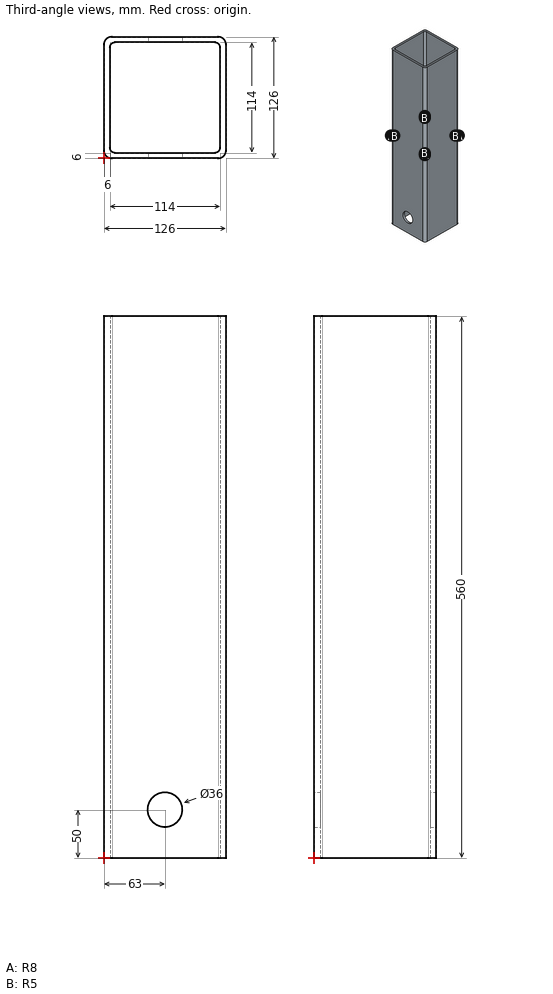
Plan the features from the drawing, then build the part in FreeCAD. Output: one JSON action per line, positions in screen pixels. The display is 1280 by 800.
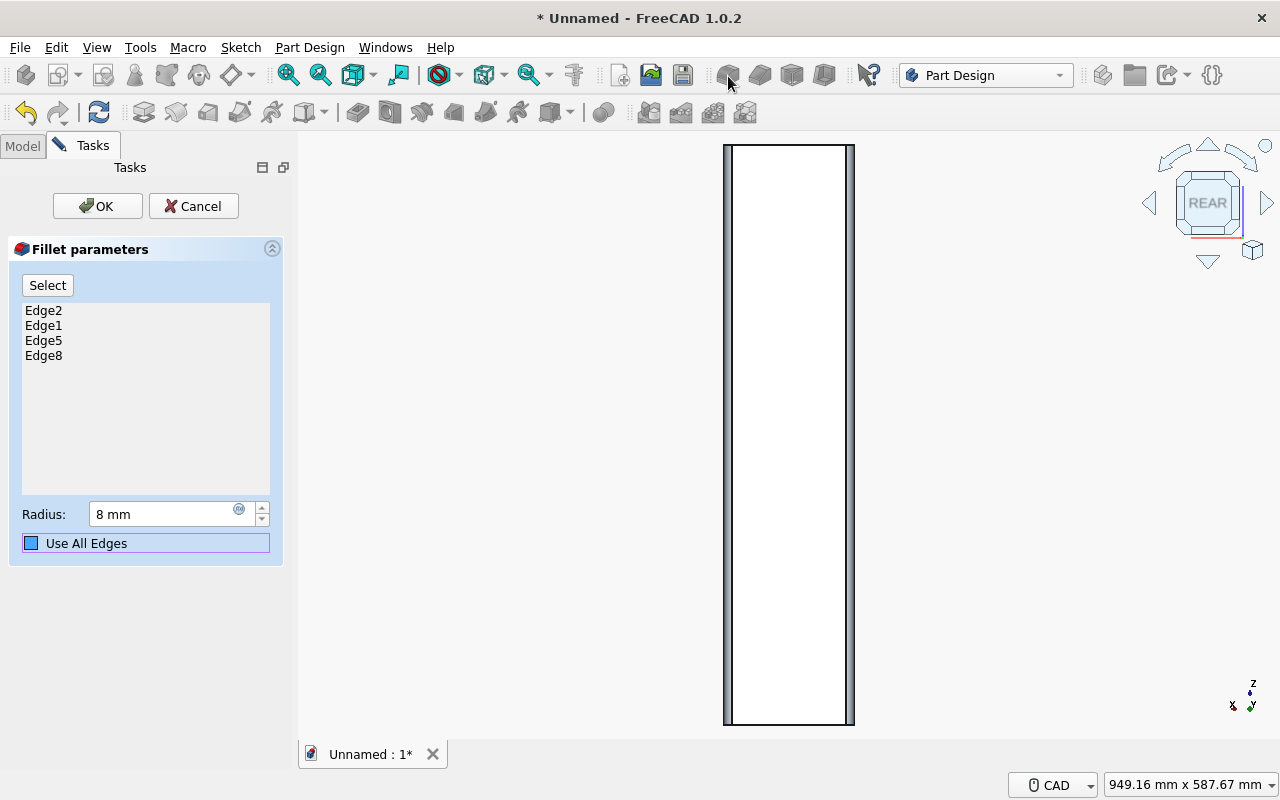
{"action": "left_click", "coordinate": [98, 206]}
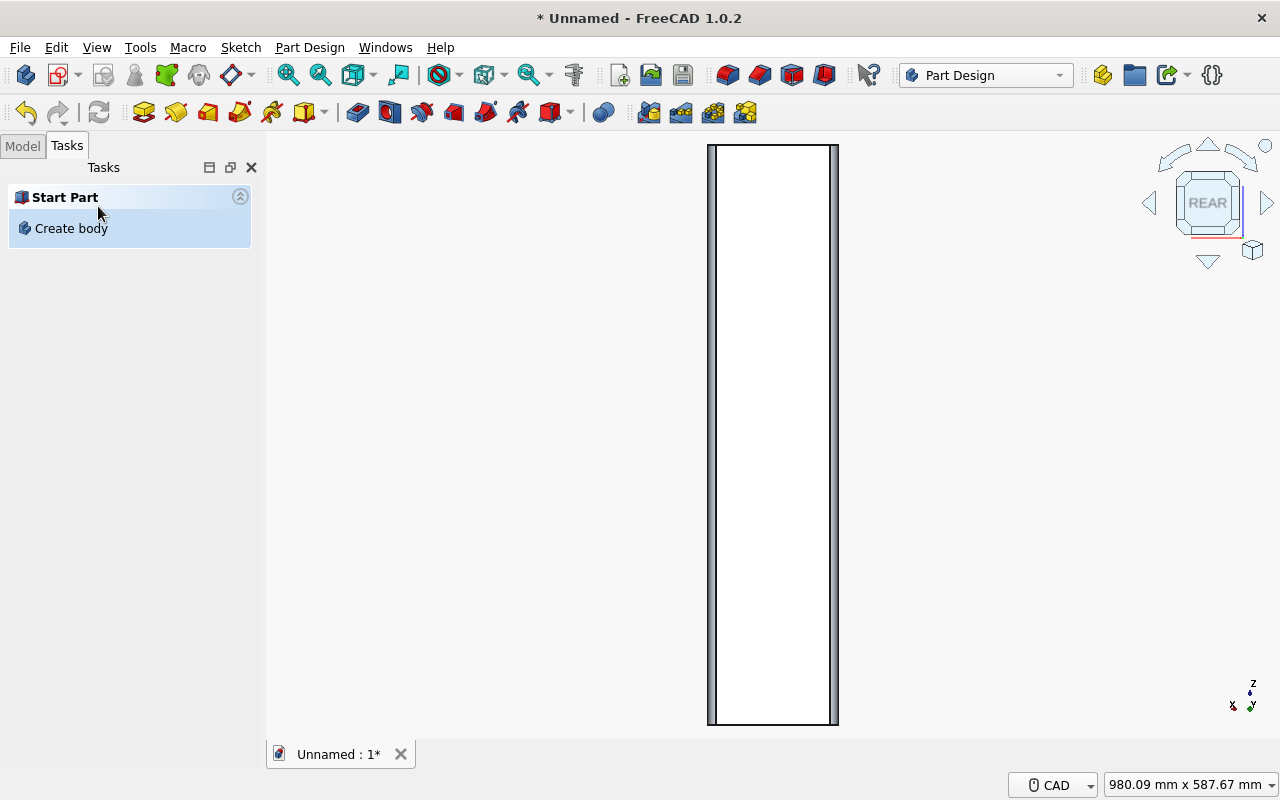
{"action": "key", "text": "0"}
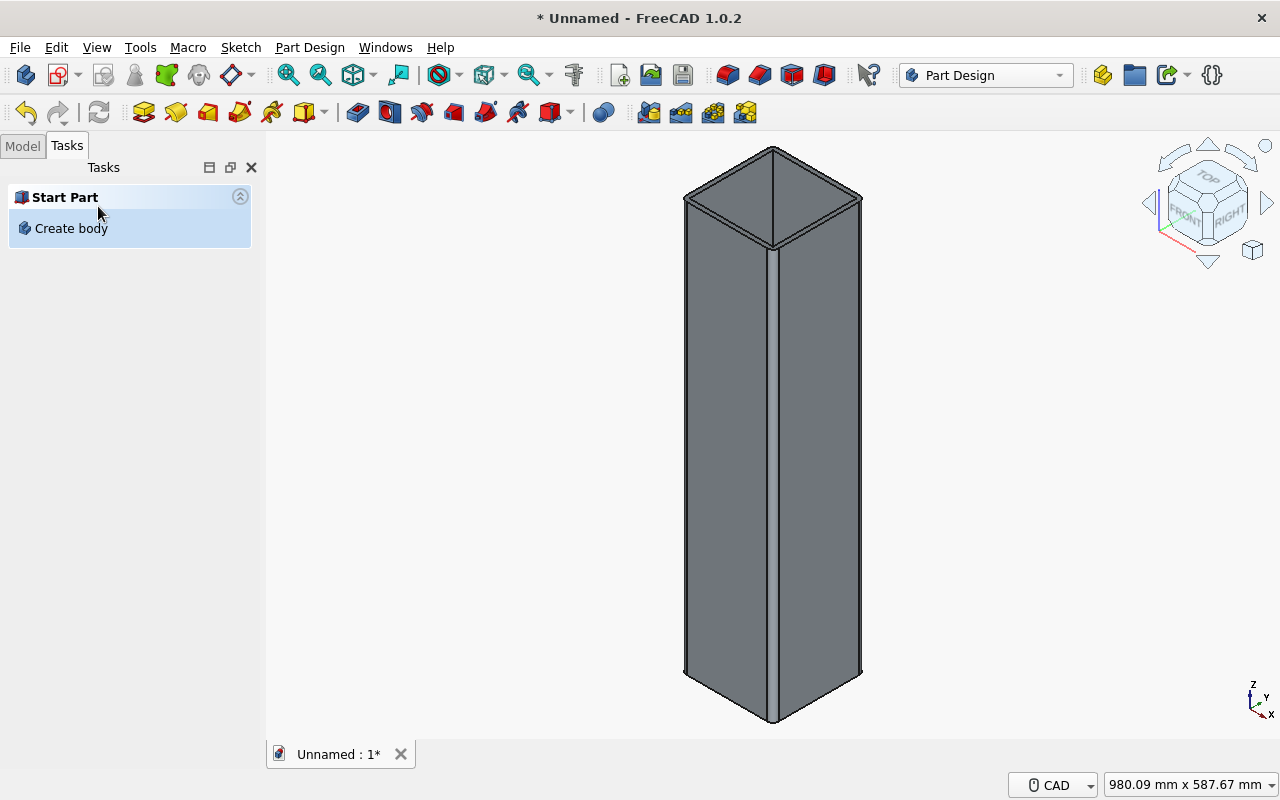
{"action": "key", "text": "2"}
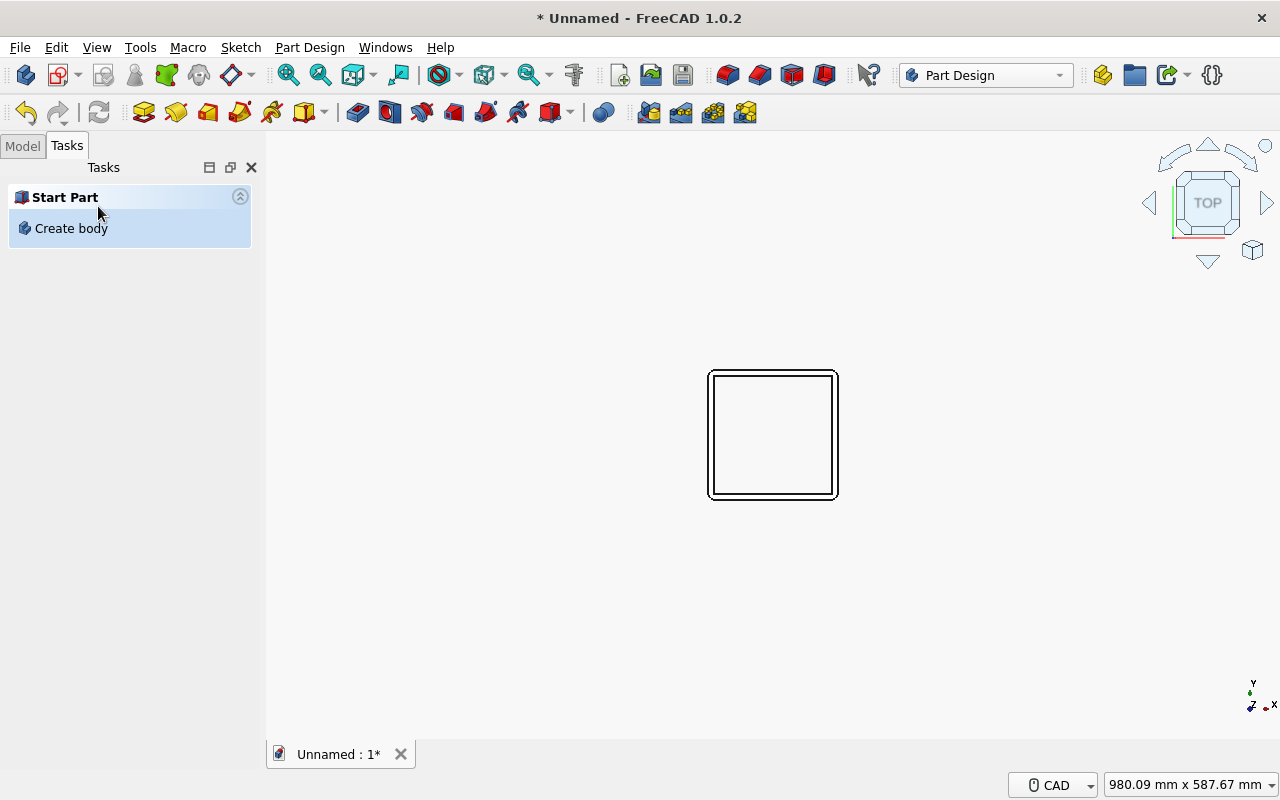
{"action": "left_click", "coordinate": [290, 76]}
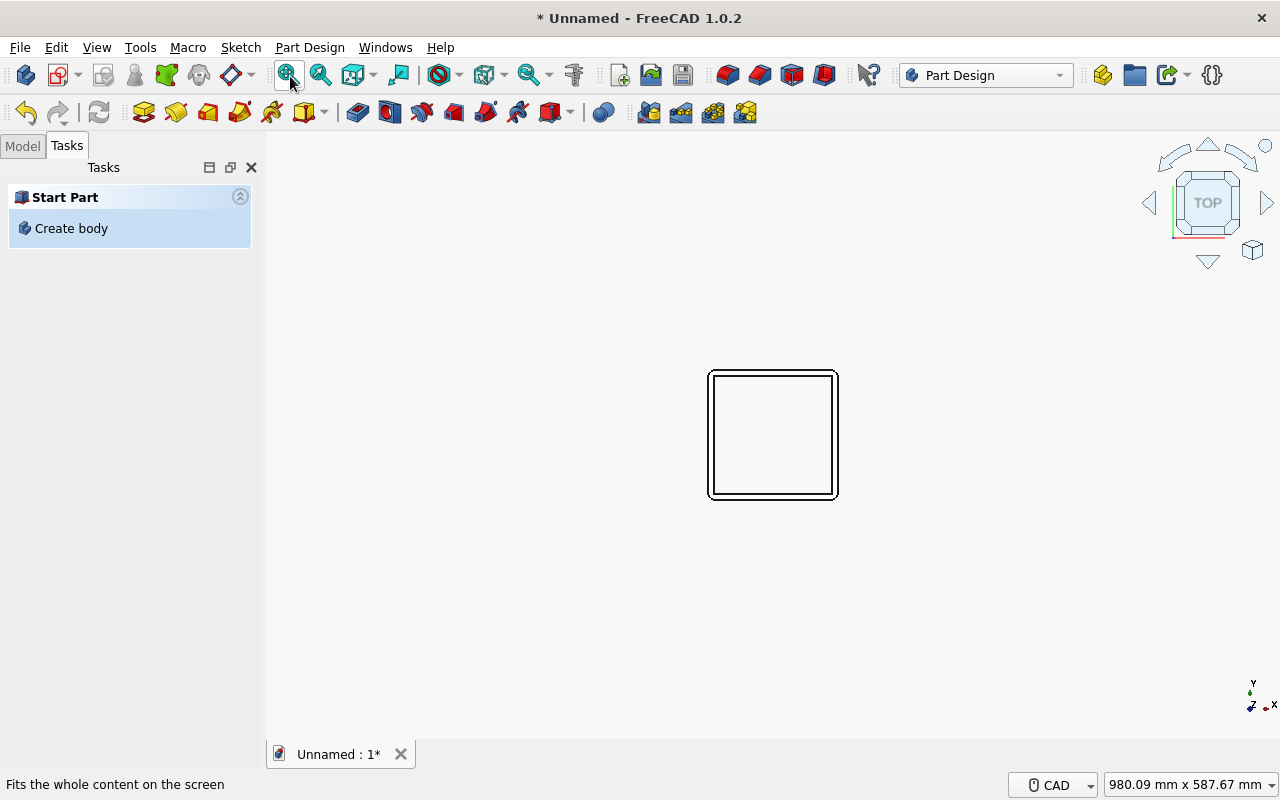
{"action": "key", "text": "1"}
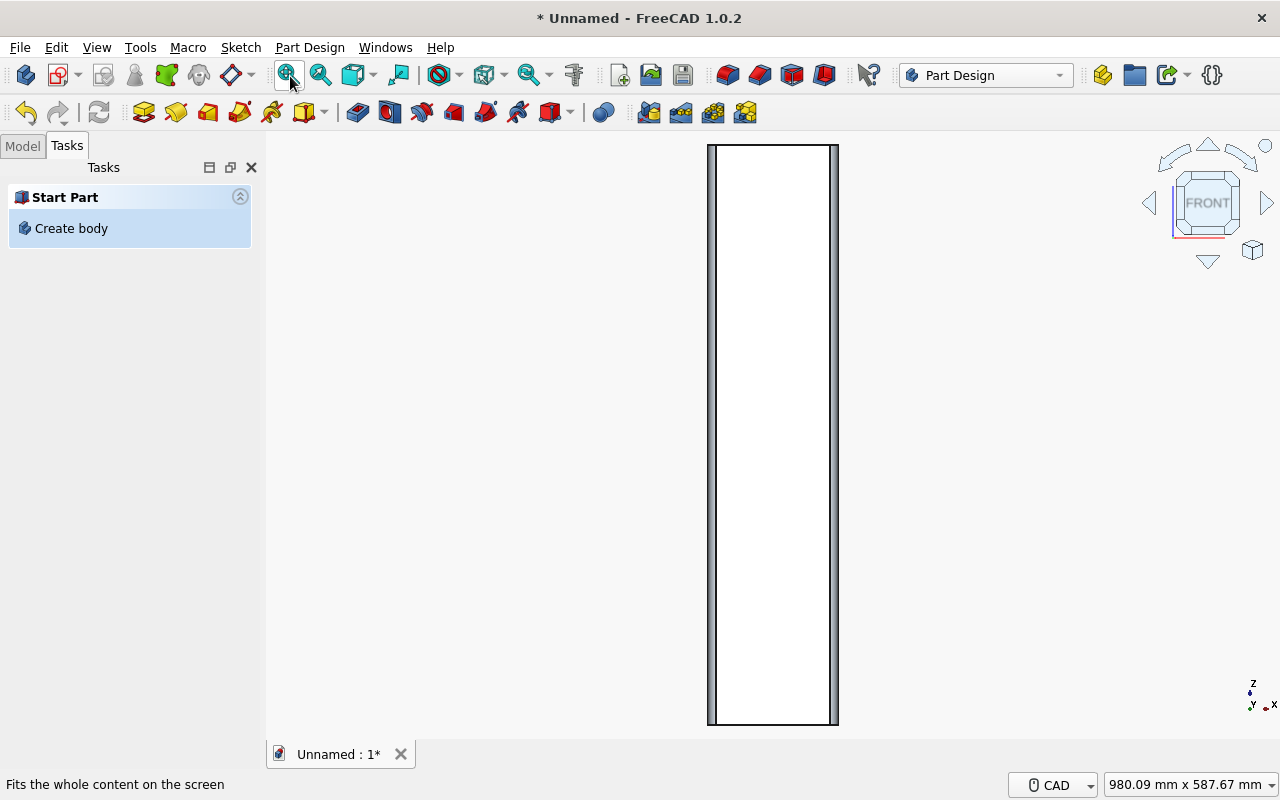
{"action": "key", "text": "3"}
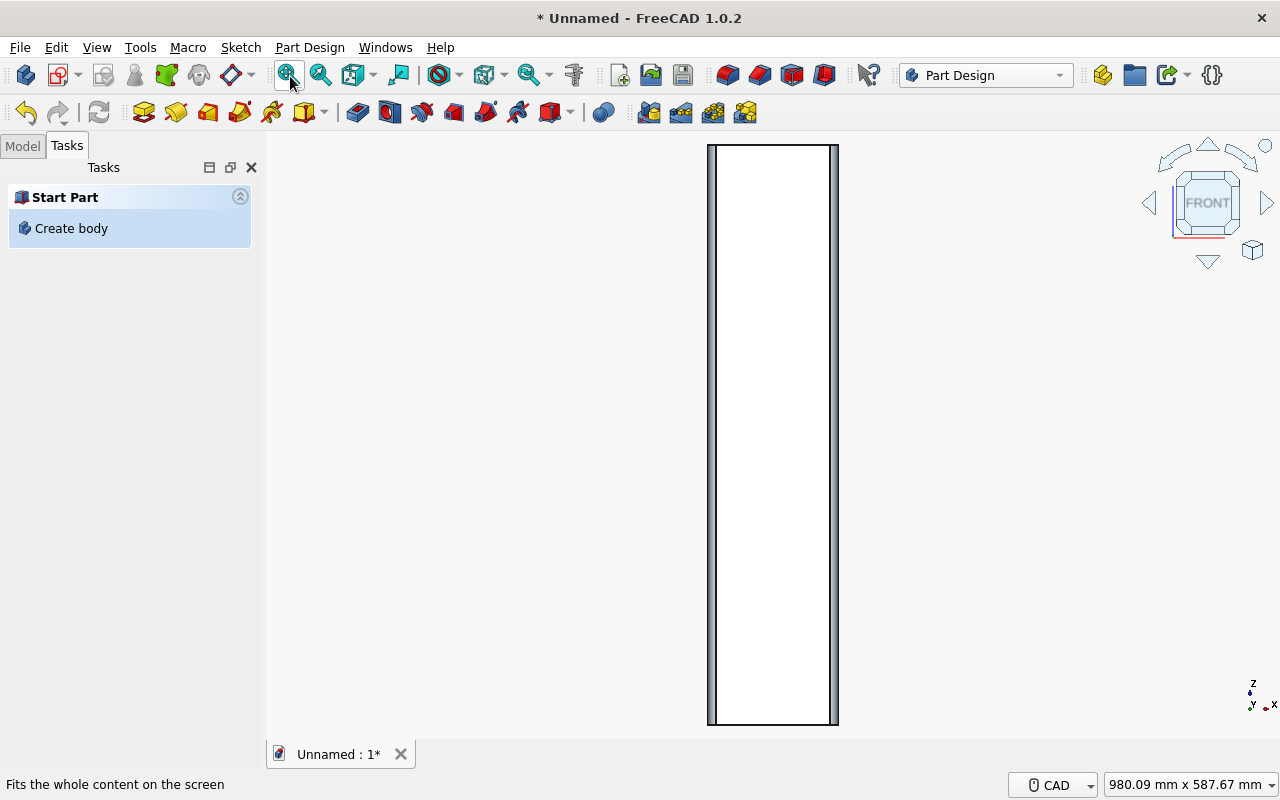
{"action": "key", "text": "5"}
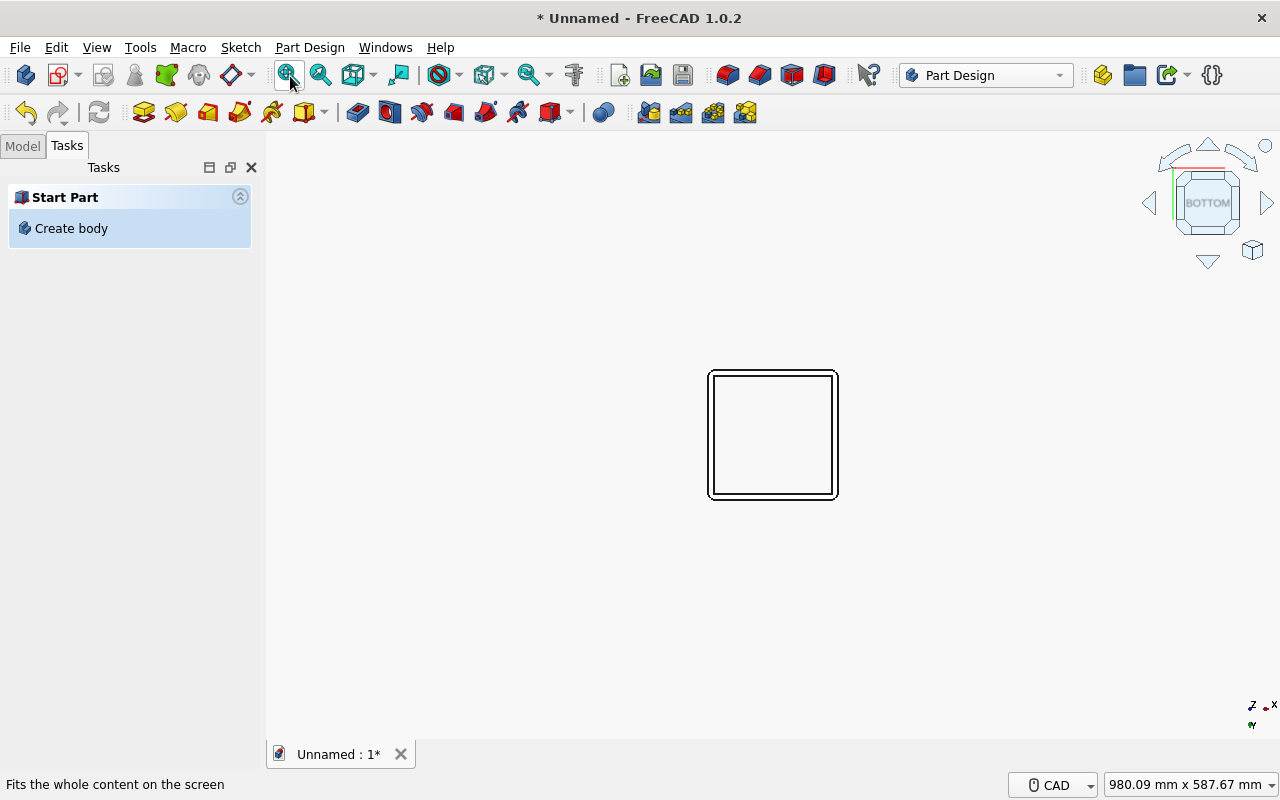
{"action": "left_click", "coordinate": [290, 76]}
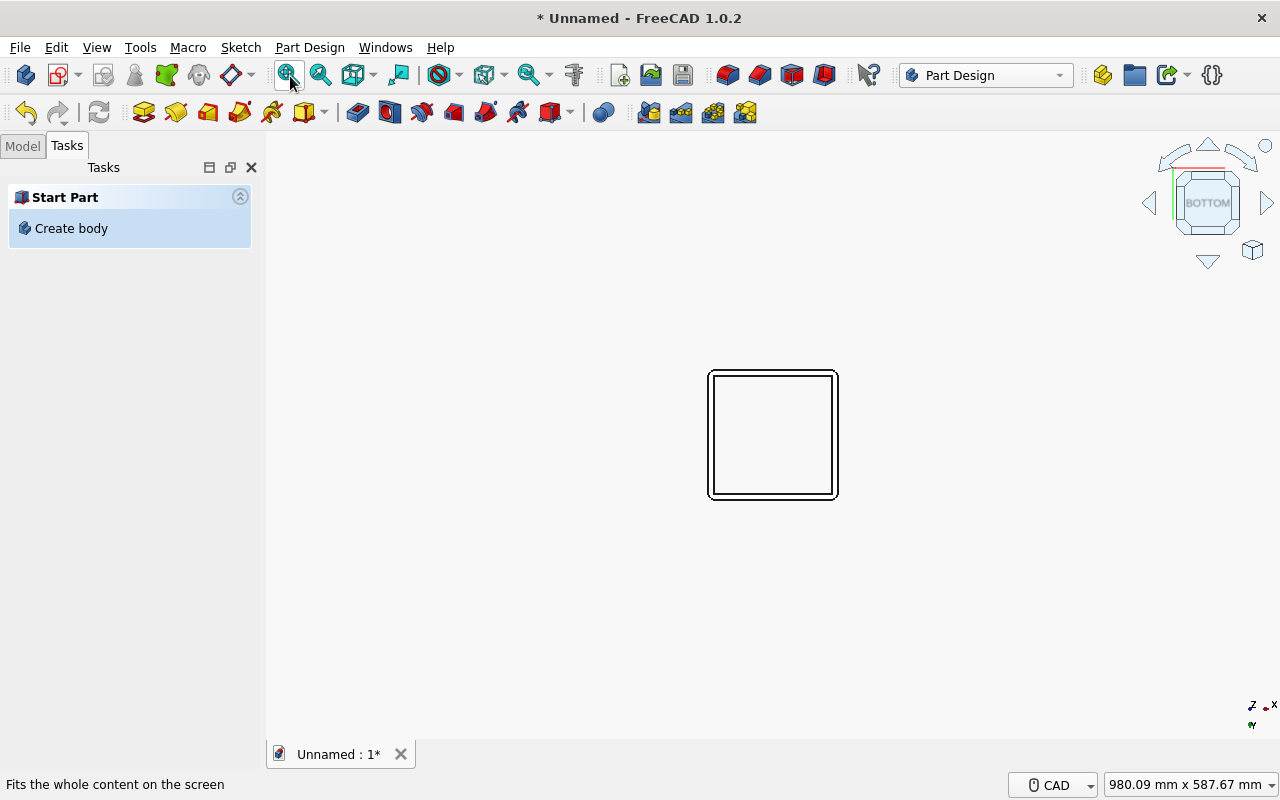
{"action": "key", "text": "4"}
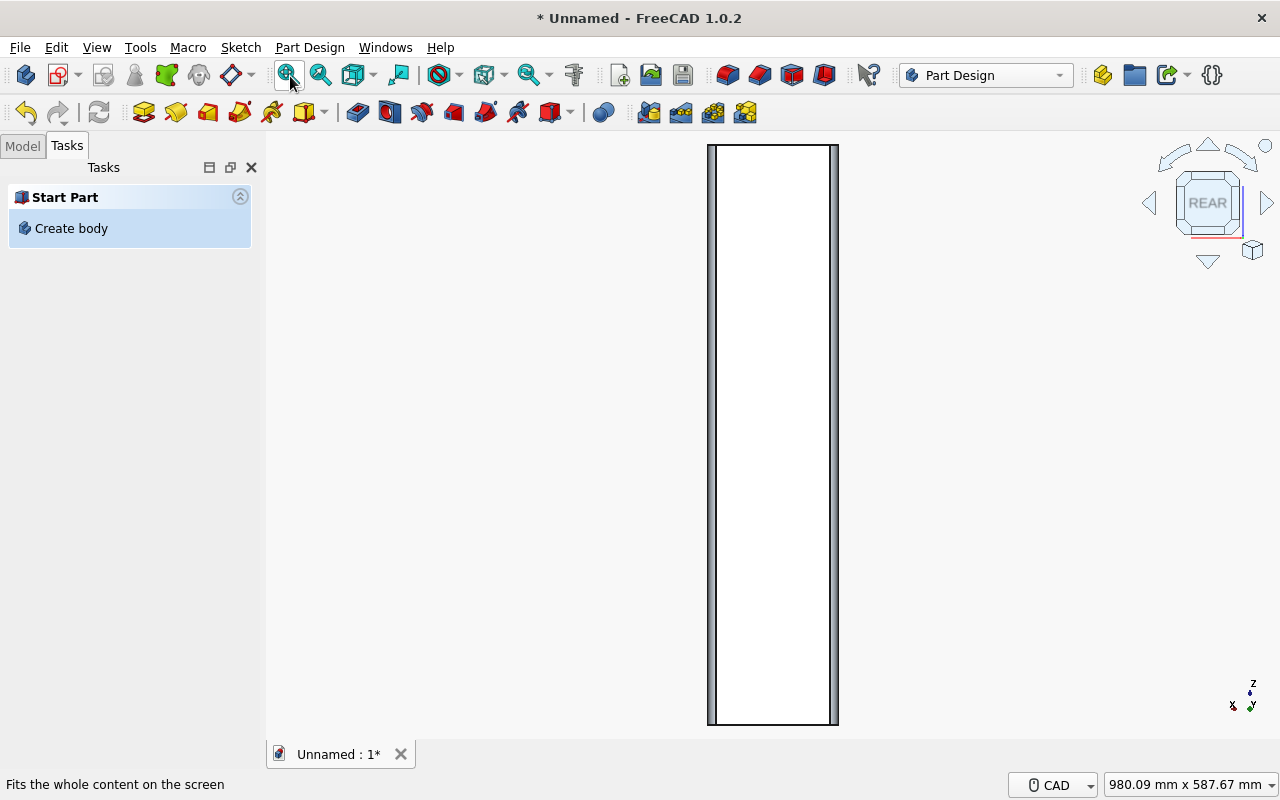
{"action": "key", "text": "6"}